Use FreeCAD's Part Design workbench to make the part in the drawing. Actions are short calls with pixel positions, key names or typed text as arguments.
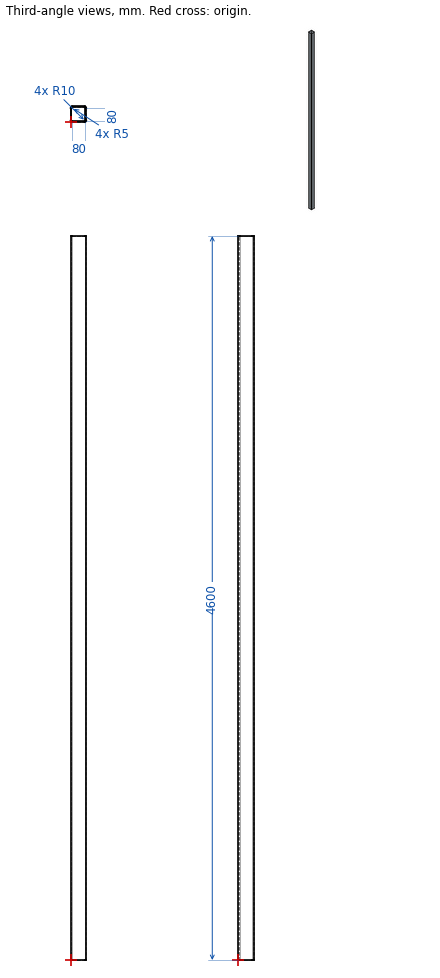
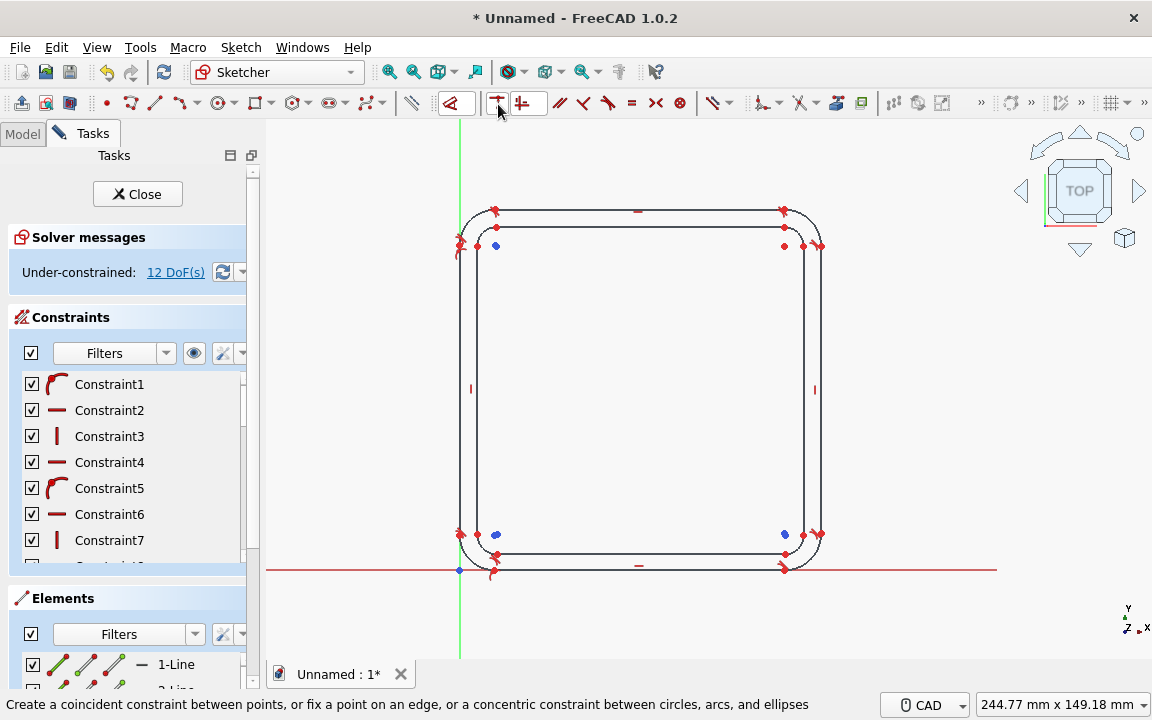
click(801, 566)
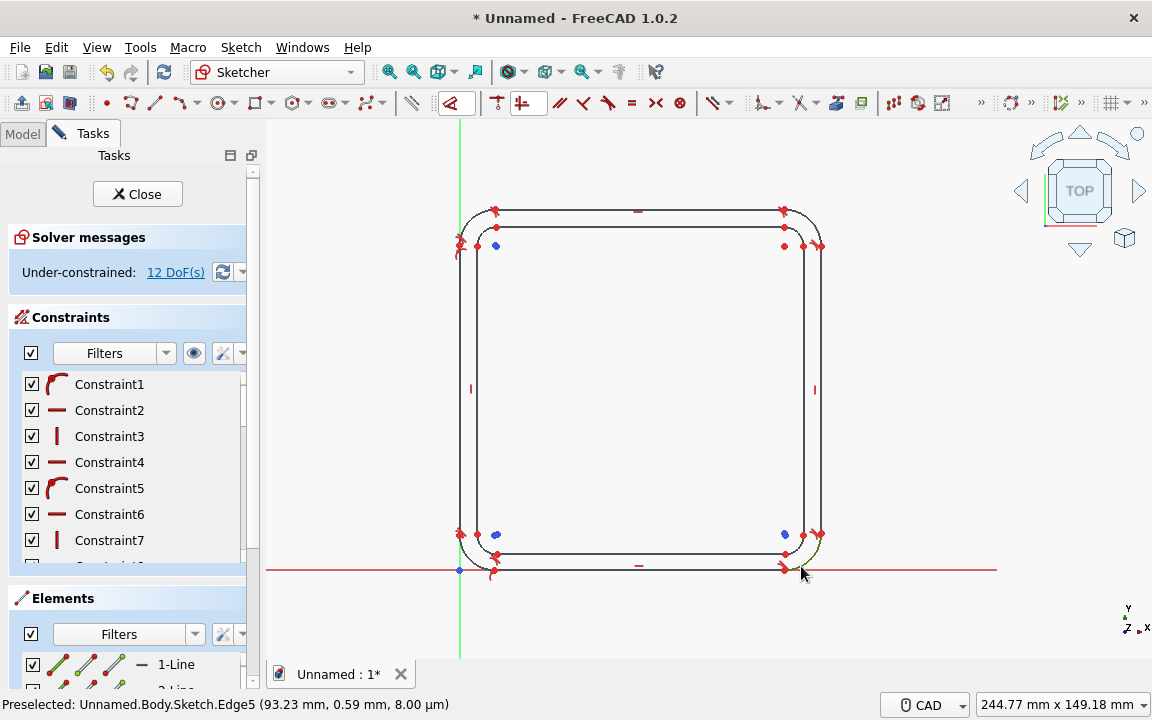
click(798, 549)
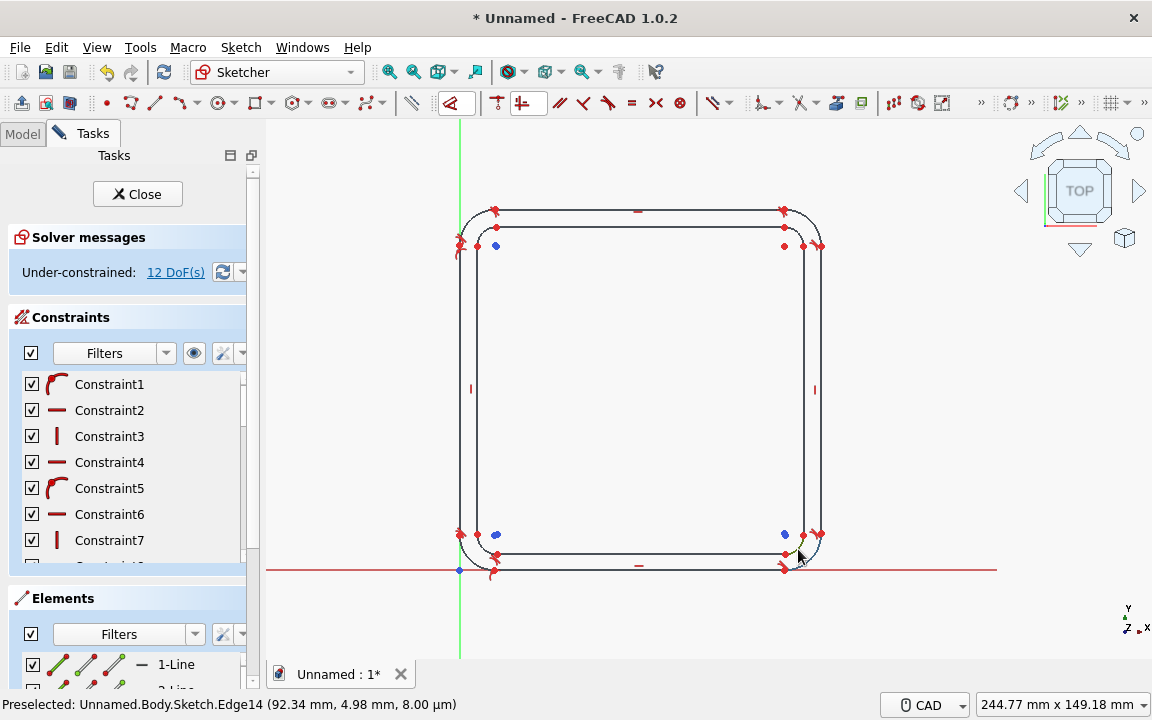
click(498, 104)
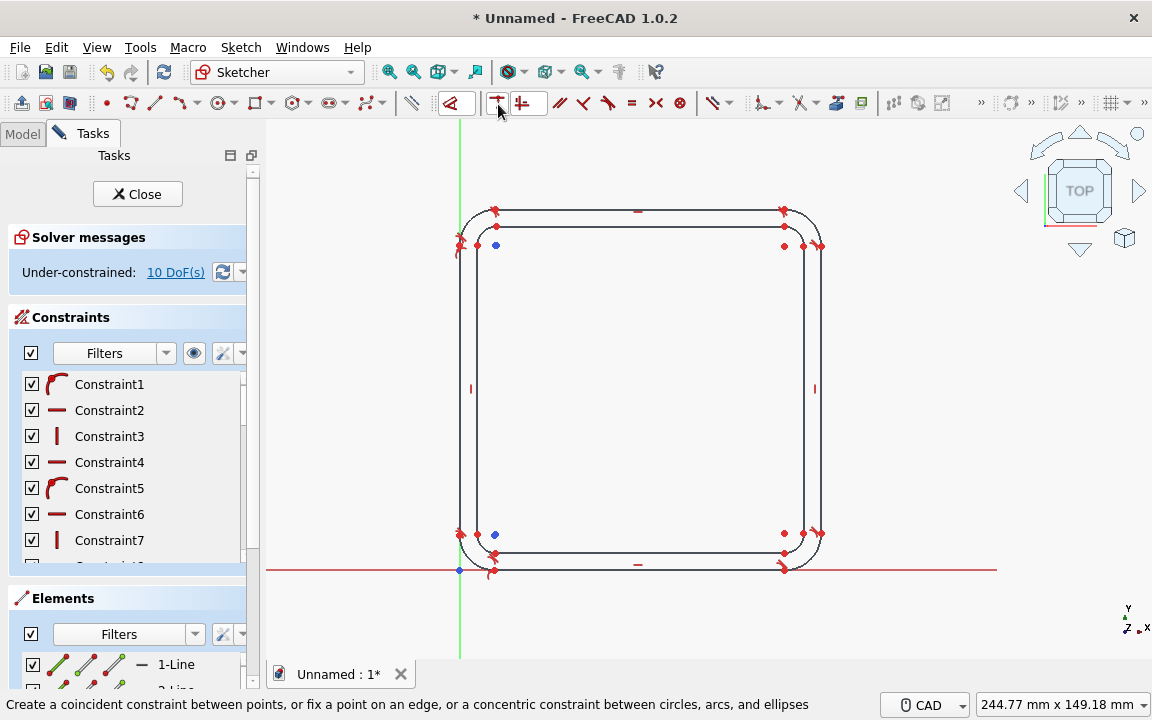
click(464, 551)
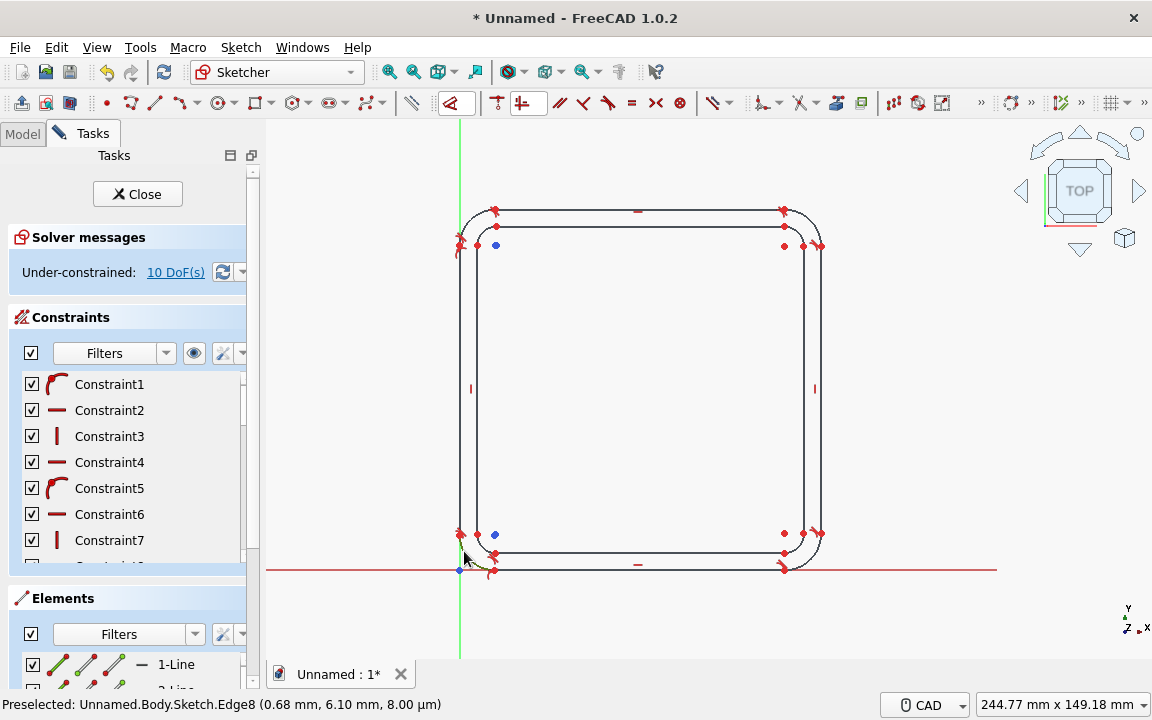
click(483, 548)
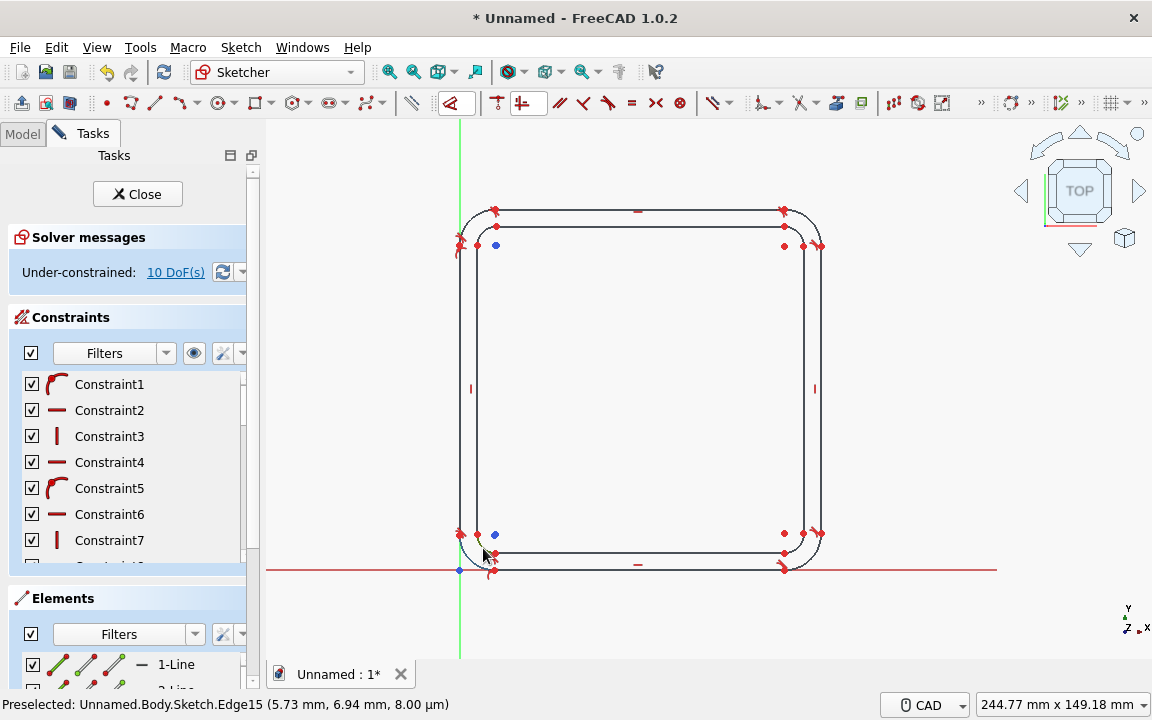
click(498, 104)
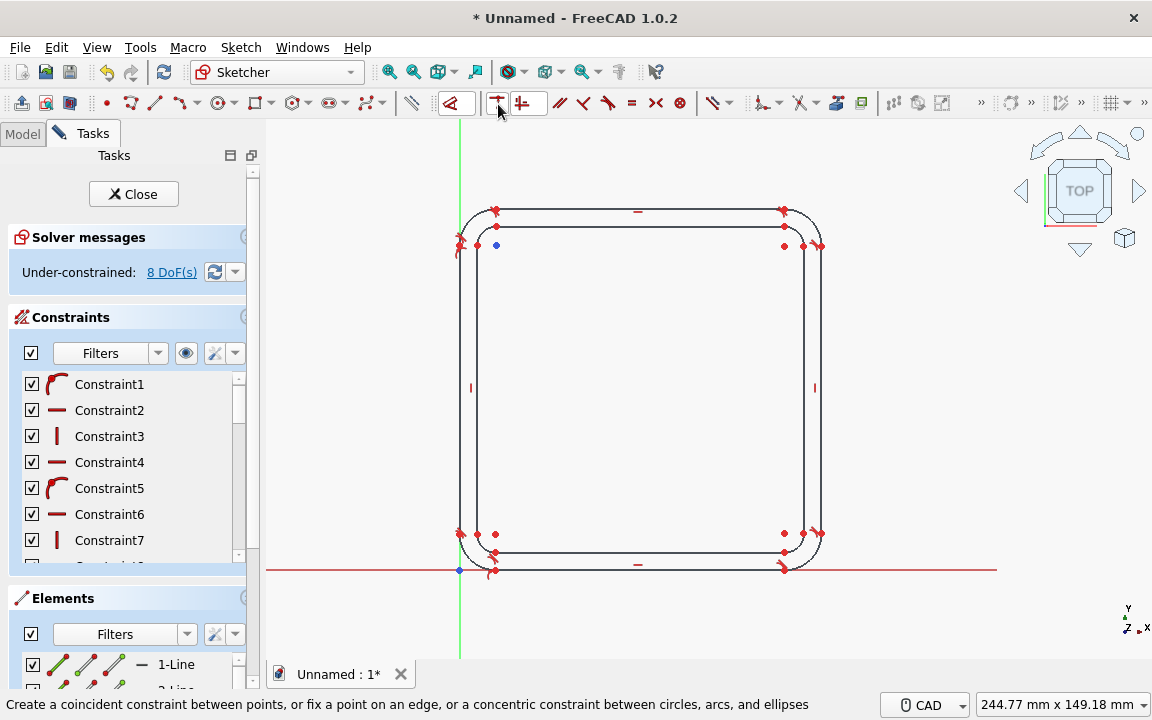
click(802, 566)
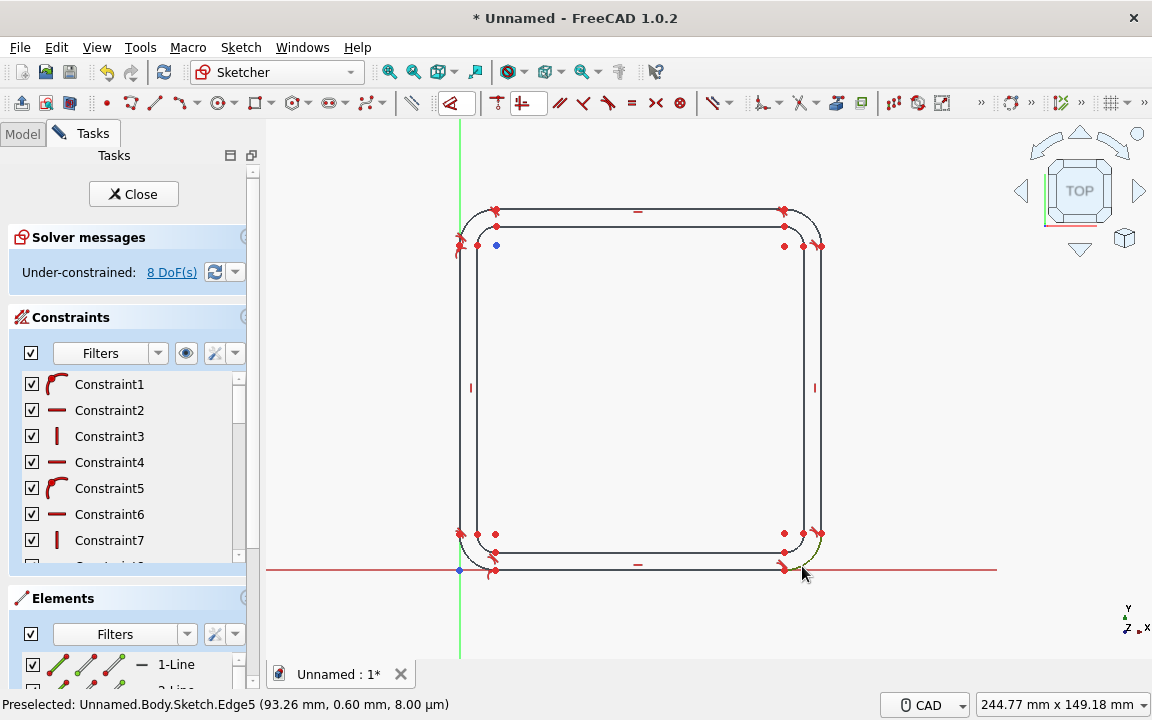
click(817, 230)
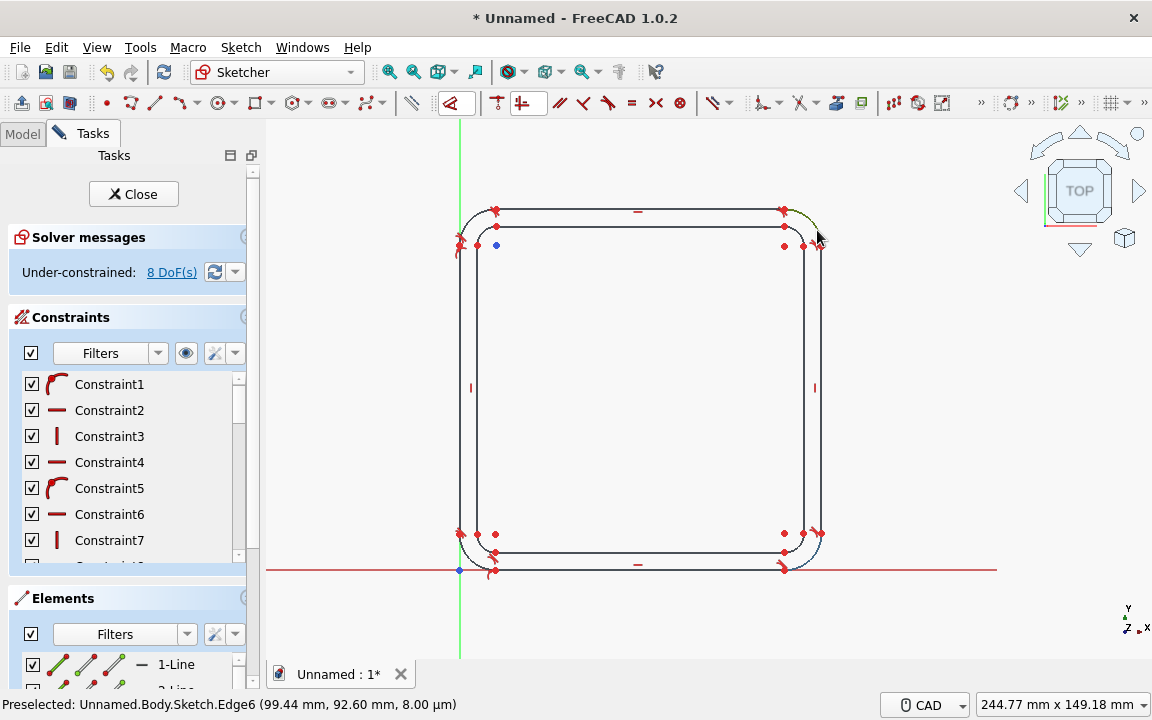
click(480, 213)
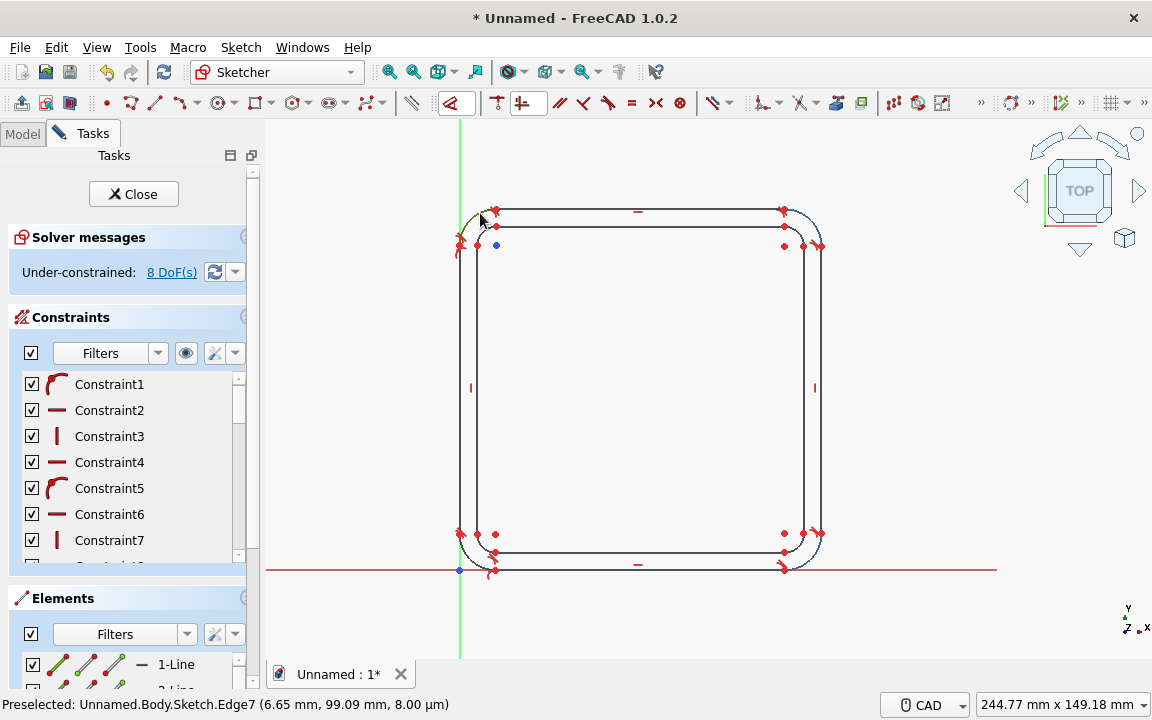
click(464, 550)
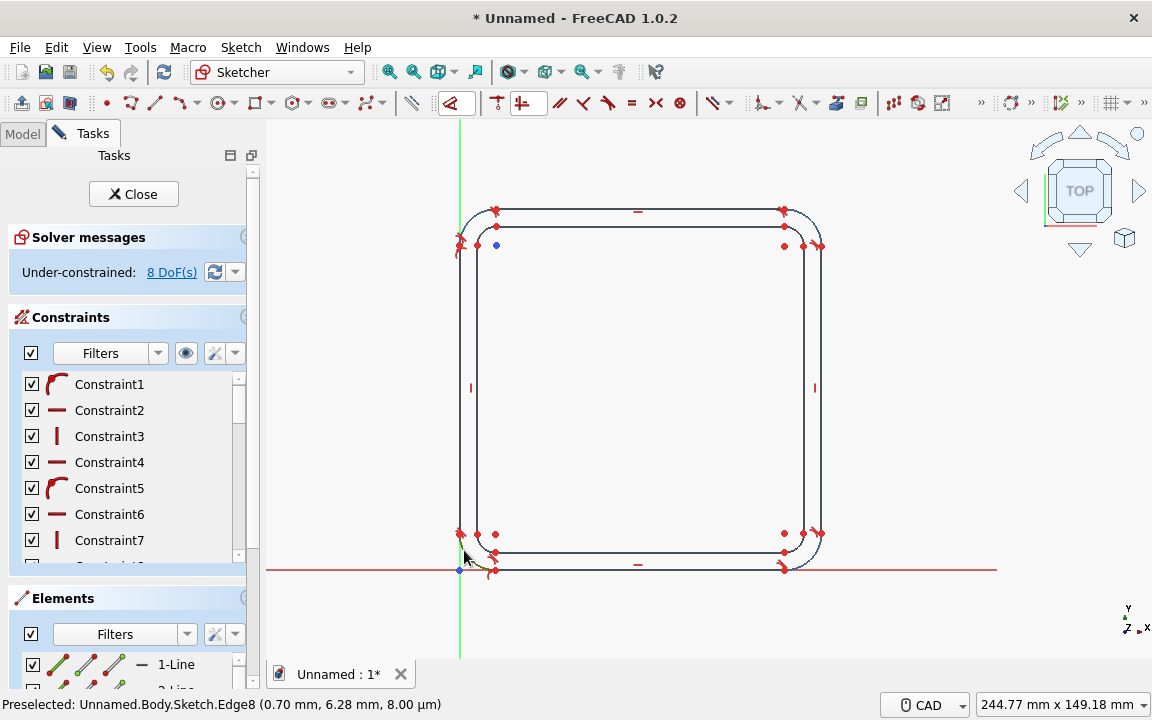
click(632, 104)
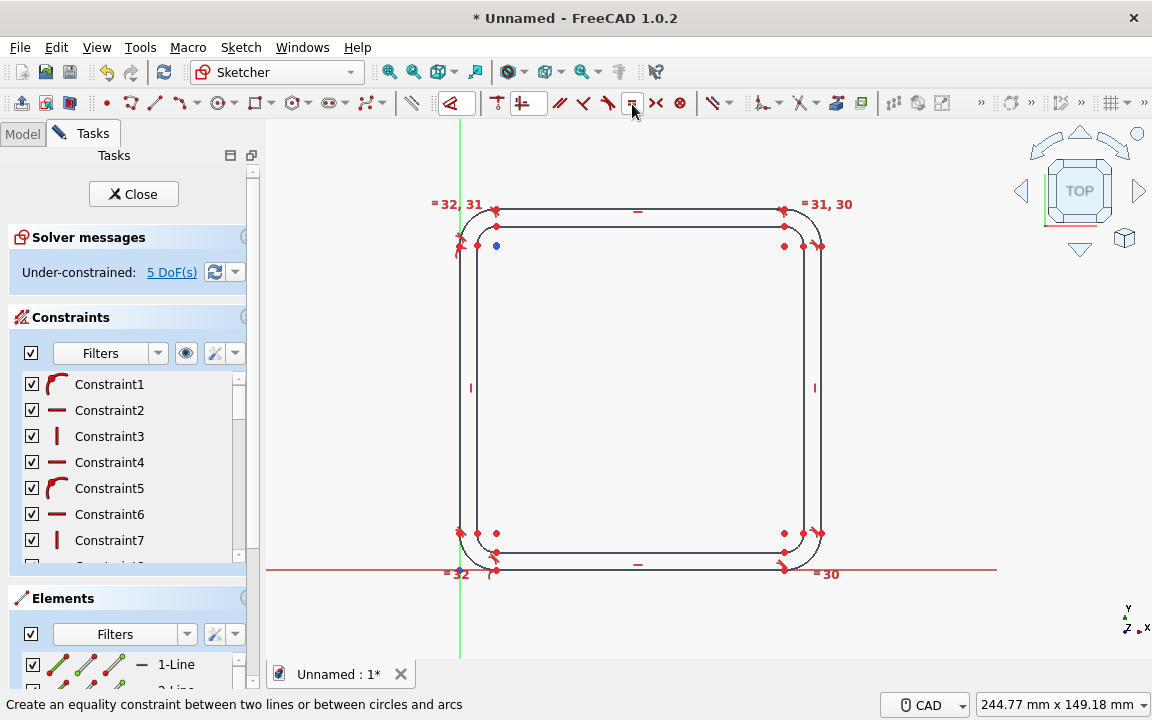
scroll(802, 237, up, 3)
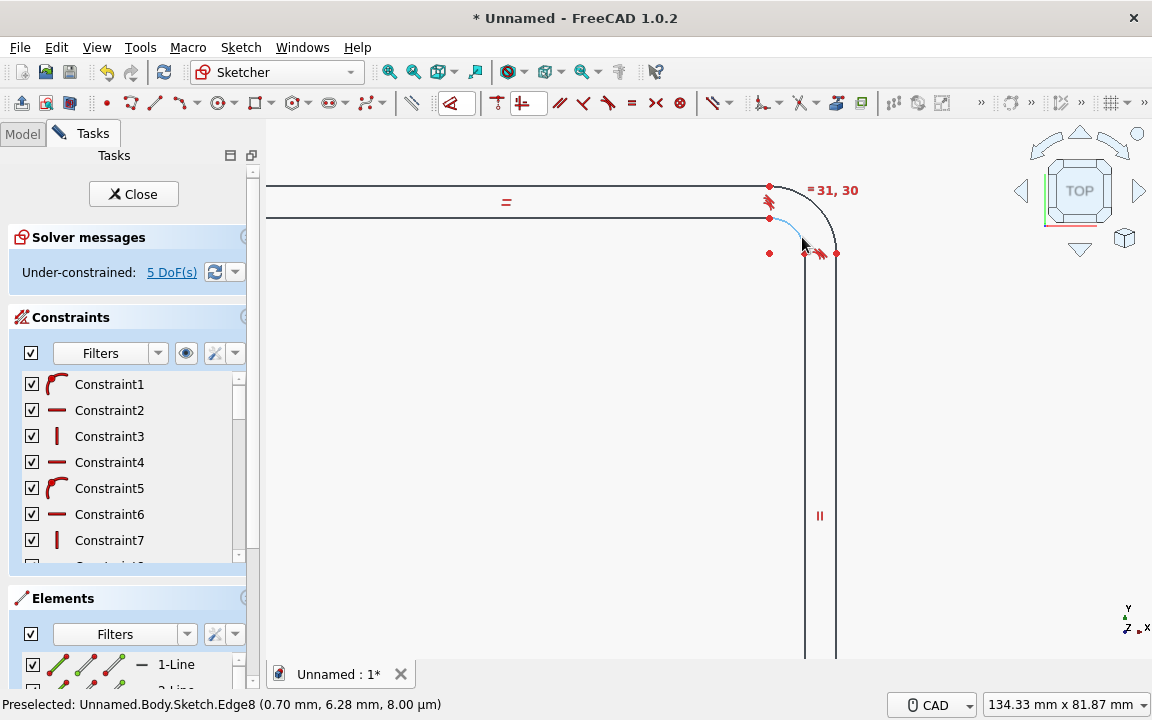
click(801, 237)